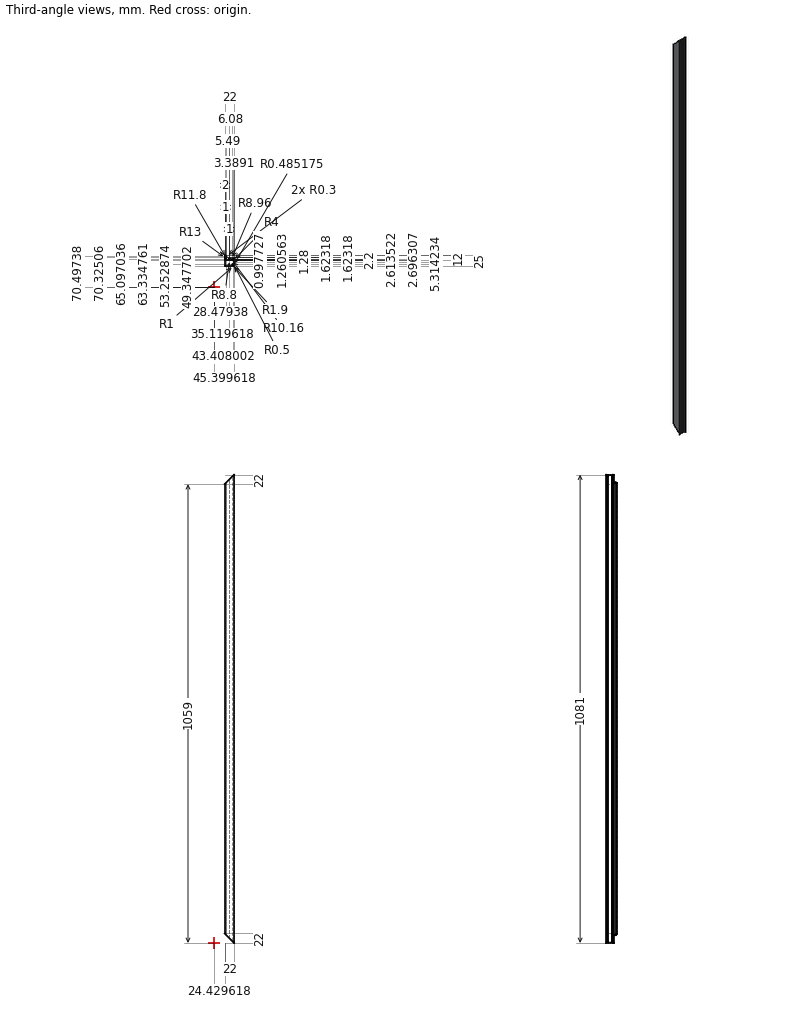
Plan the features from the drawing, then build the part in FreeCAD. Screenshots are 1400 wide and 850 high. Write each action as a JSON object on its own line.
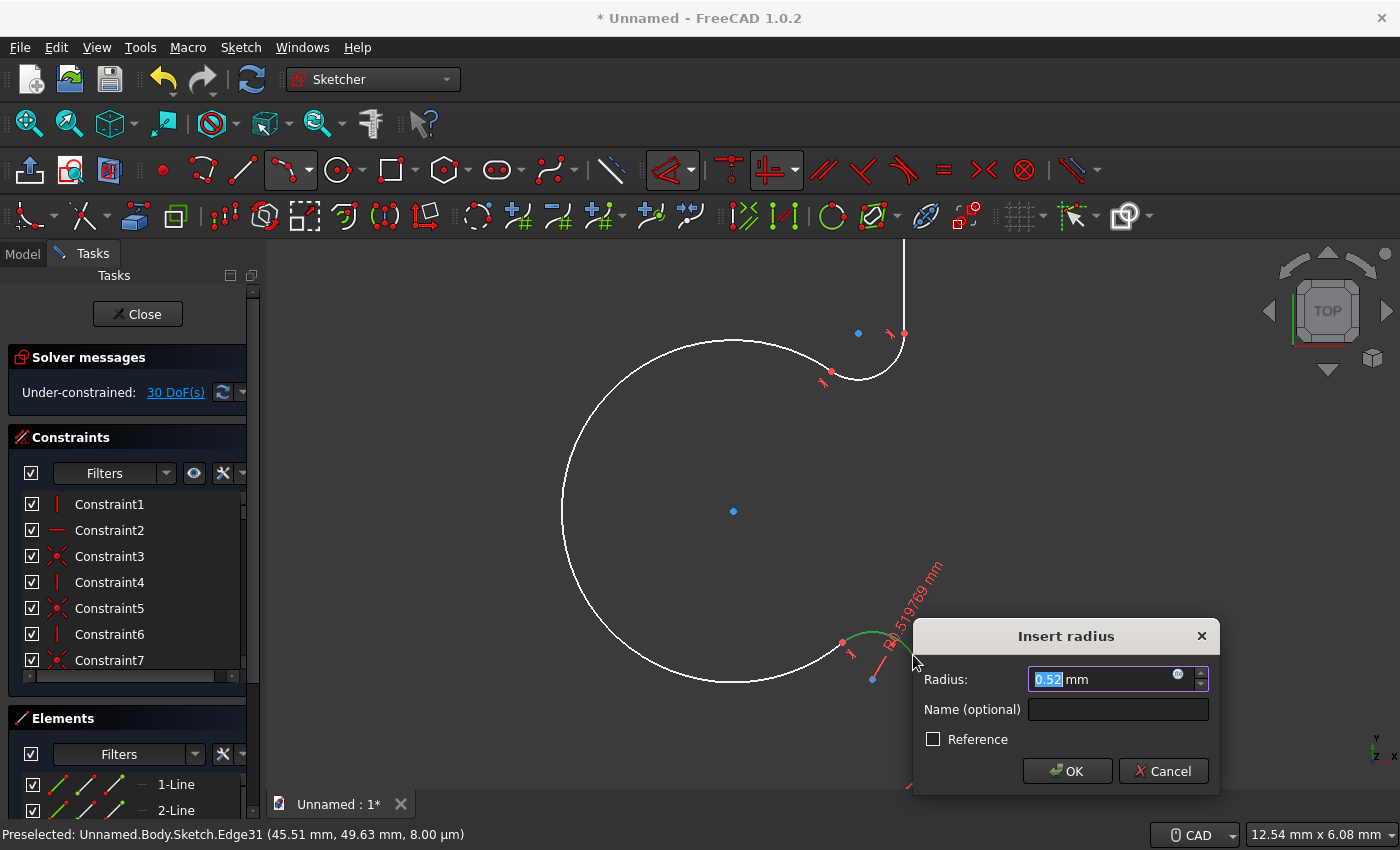
{"action": "type", "text": "0.485175"}
{"action": "key", "text": "Return"}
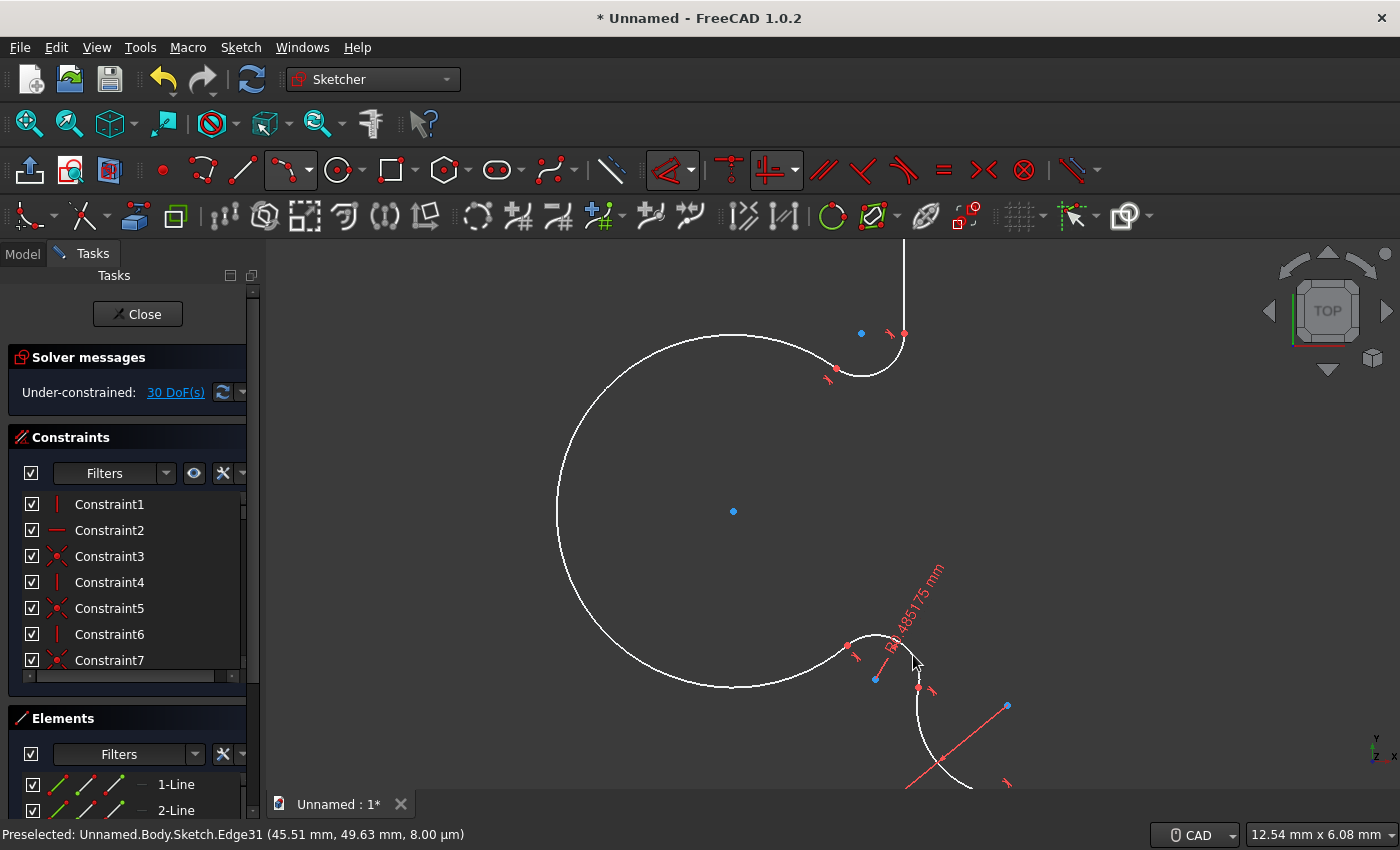
{"action": "scroll", "coordinate": [915, 684], "scroll_direction": "down", "scroll_amount": 9}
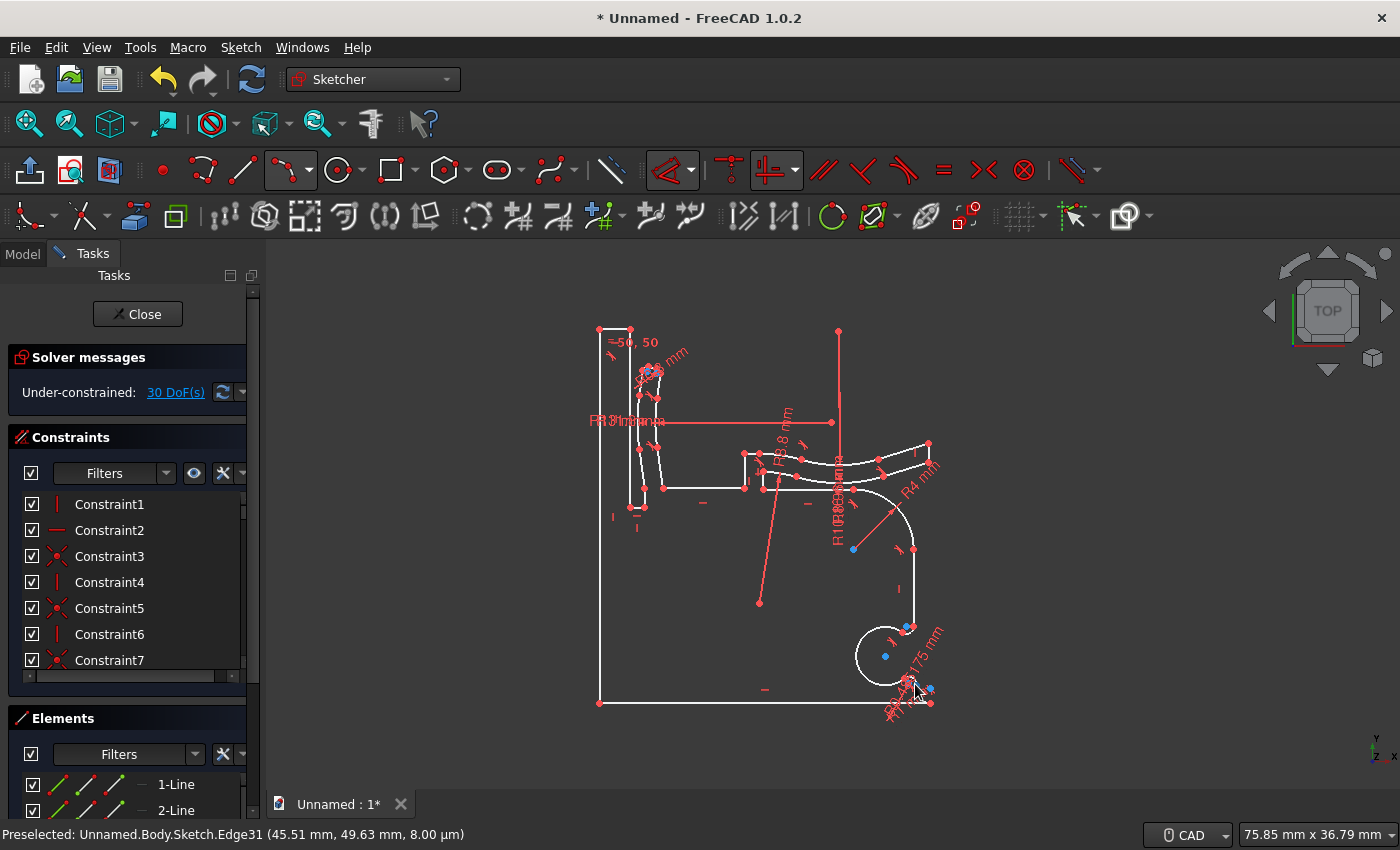
{"action": "scroll", "coordinate": [866, 634], "scroll_direction": "up", "scroll_amount": 2}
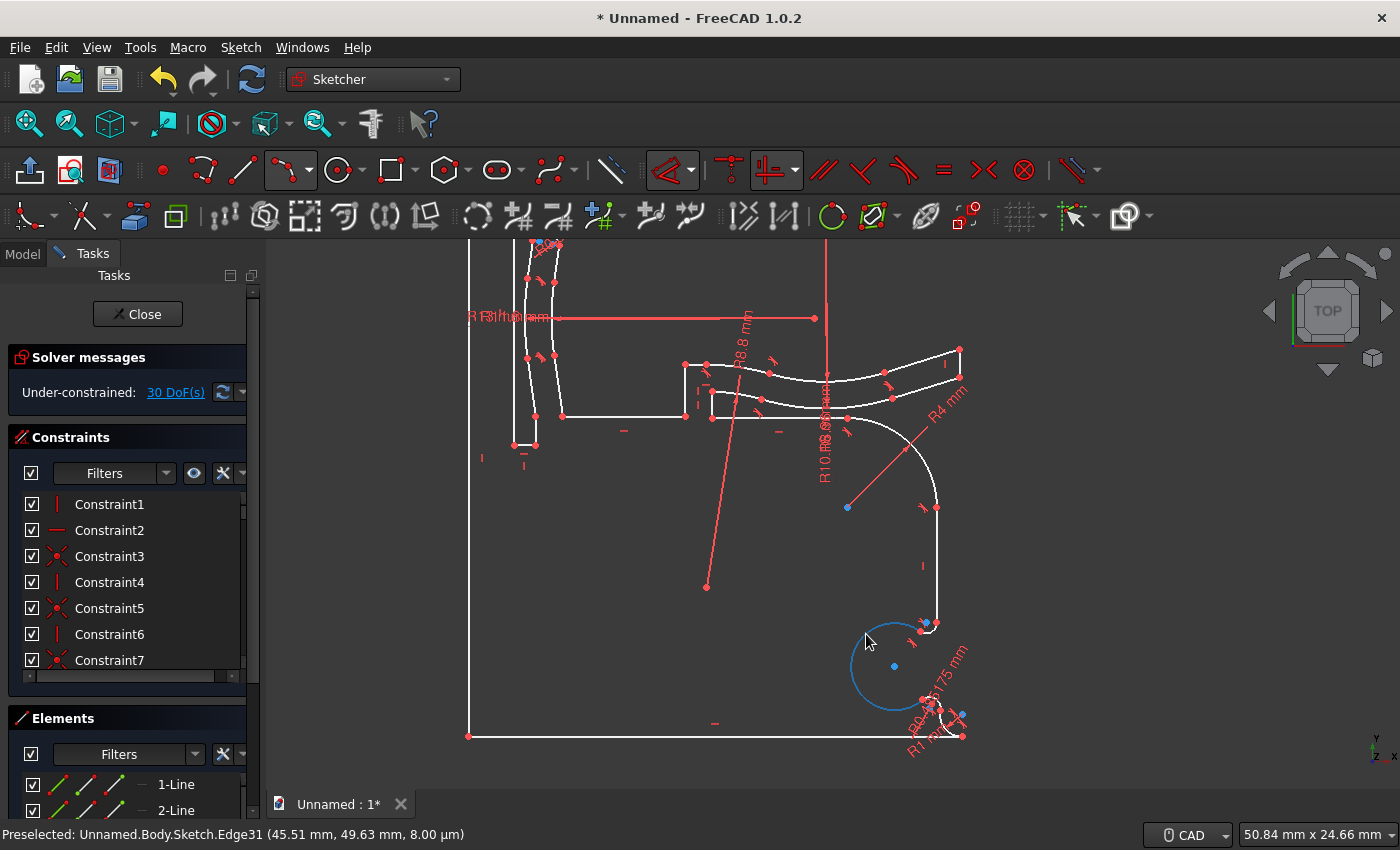
{"action": "left_click", "coordinate": [866, 634]}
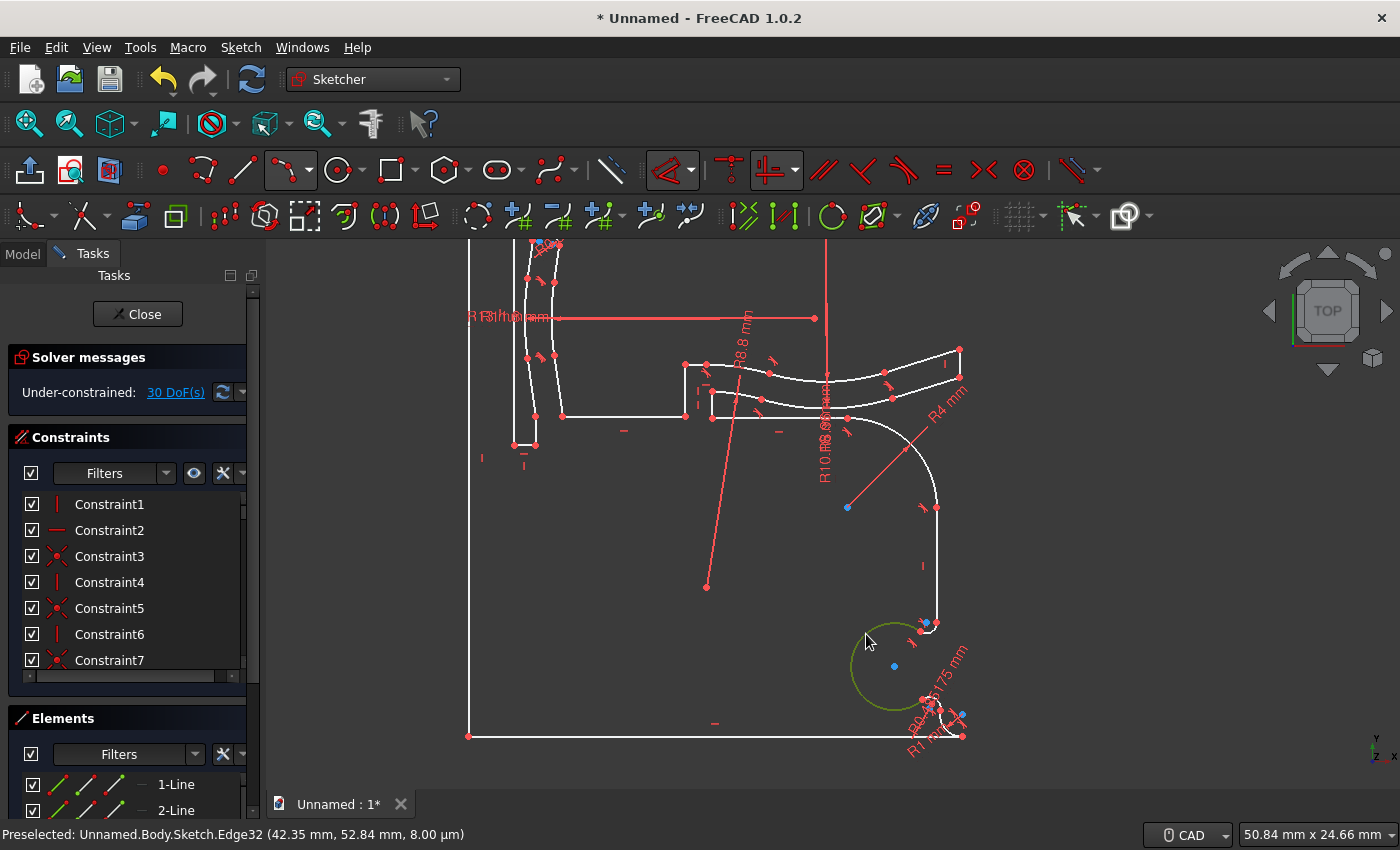
{"action": "key", "text": "k r"}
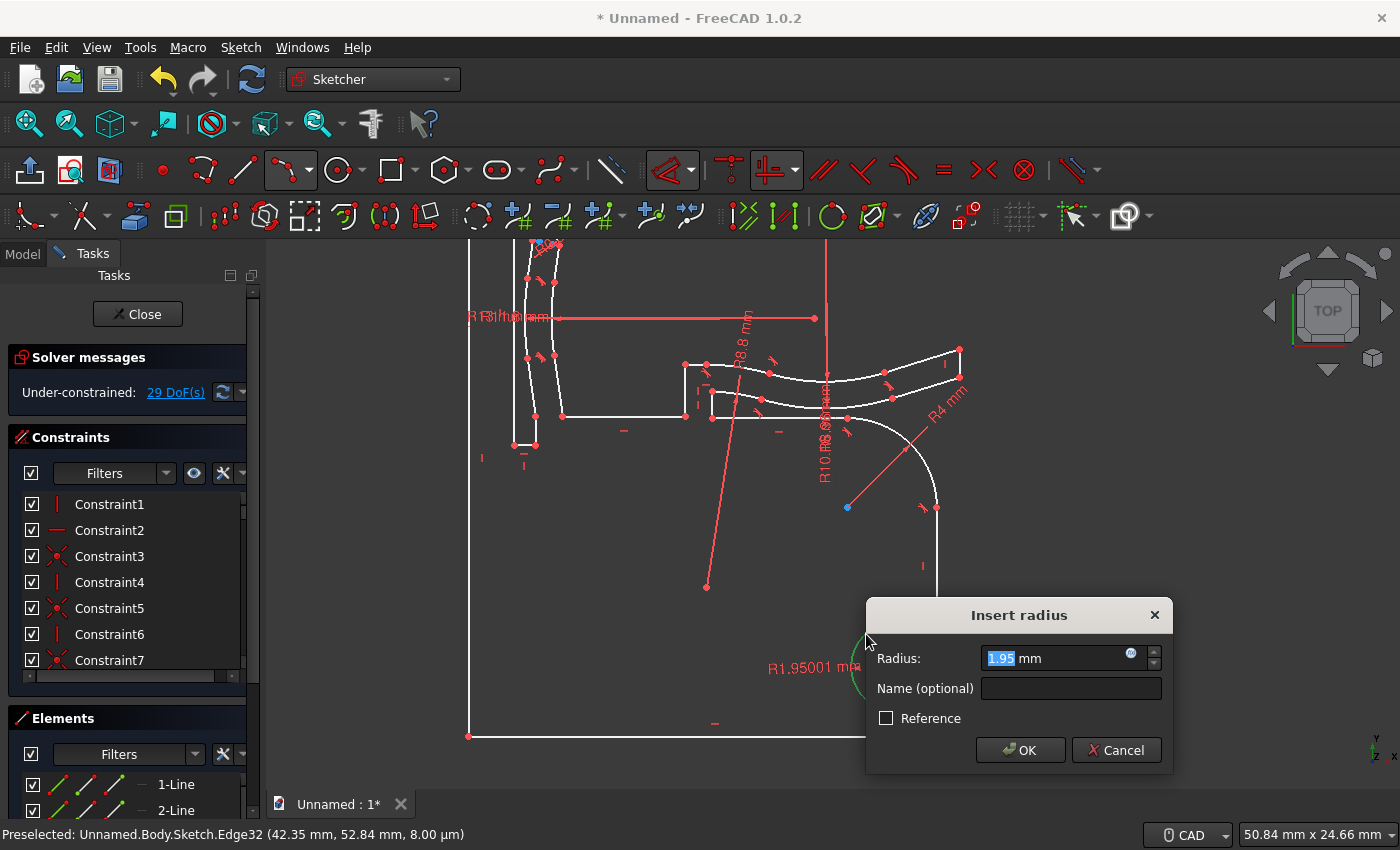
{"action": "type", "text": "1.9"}
{"action": "key", "text": "Return"}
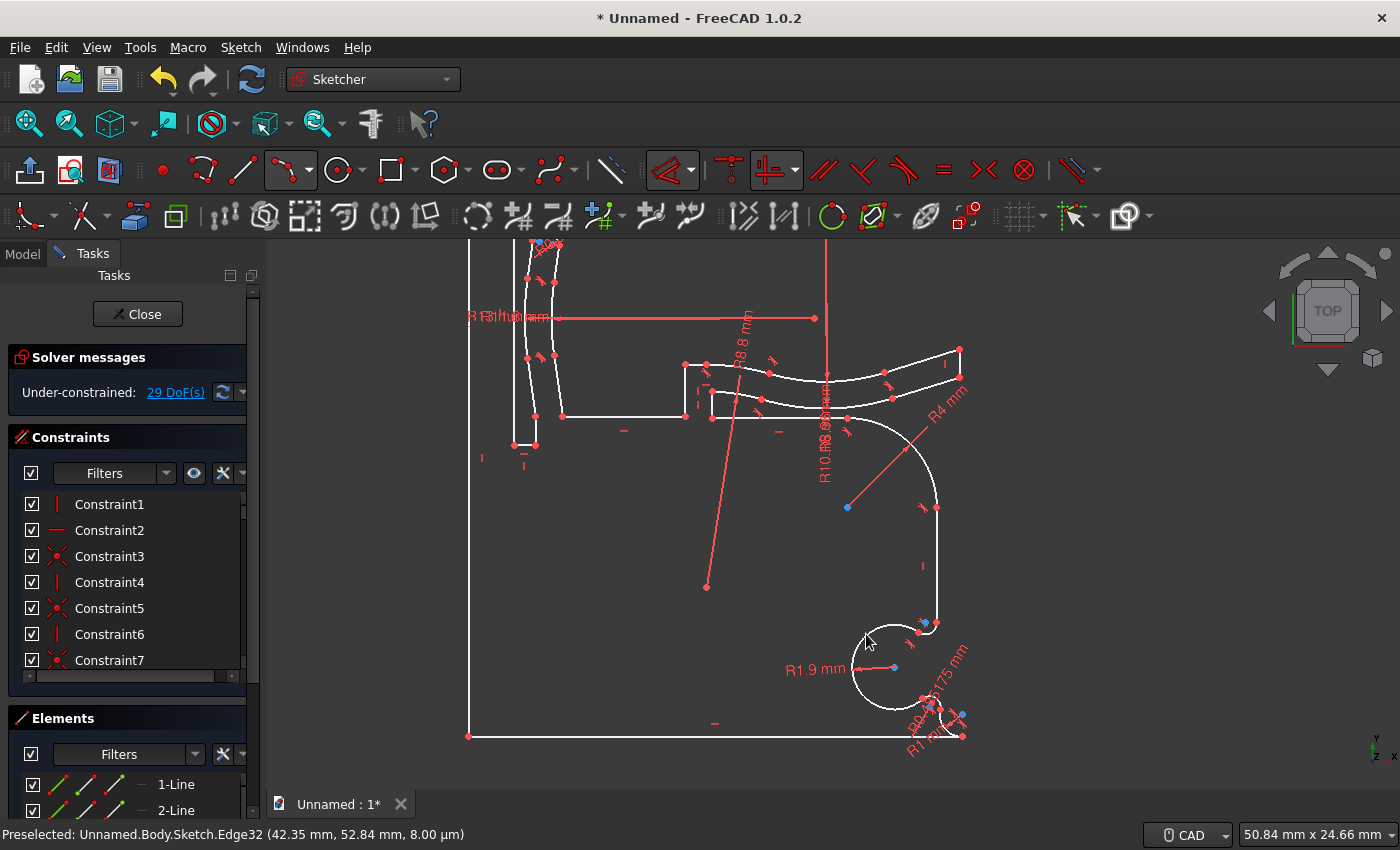
{"action": "scroll", "coordinate": [931, 633], "scroll_direction": "up", "scroll_amount": 7}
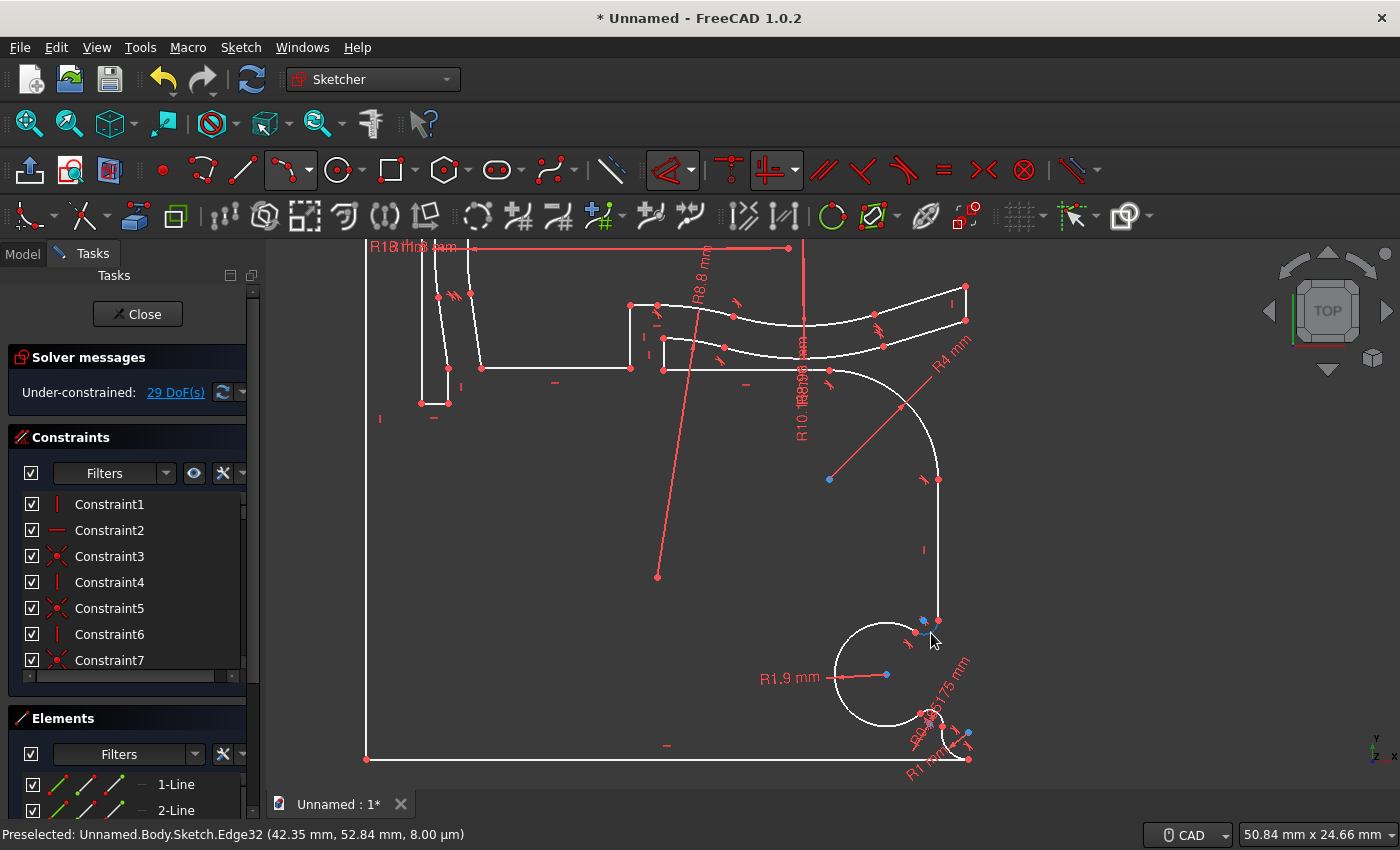
{"action": "left_click", "coordinate": [928, 631]}